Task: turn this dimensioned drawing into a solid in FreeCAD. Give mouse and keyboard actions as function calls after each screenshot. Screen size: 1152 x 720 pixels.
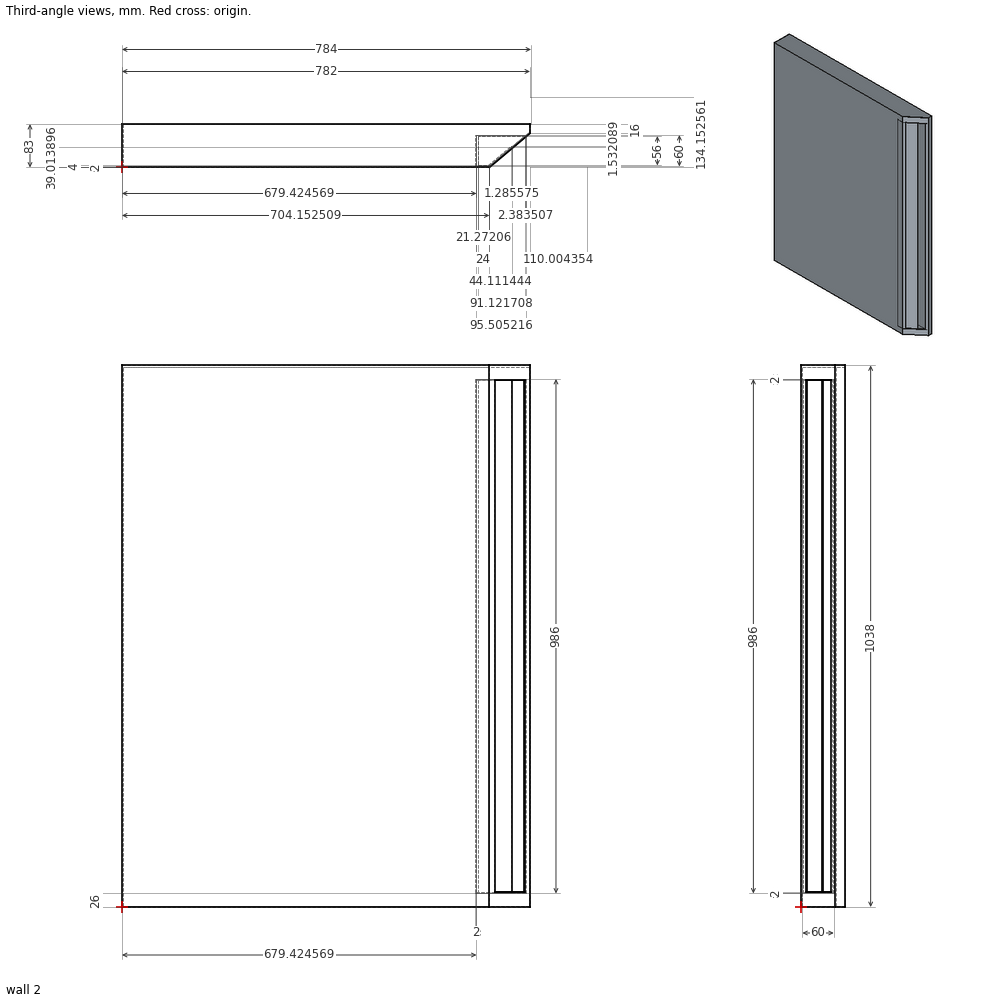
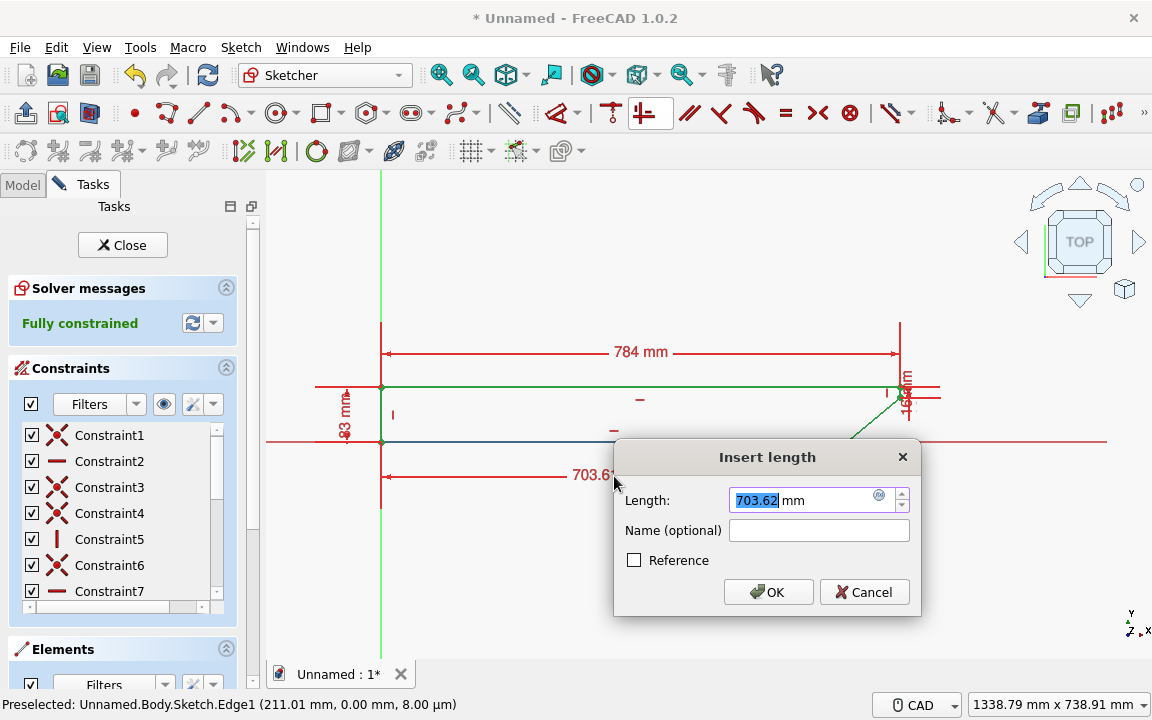
text(704.152509)
key(Return)
key(Escape)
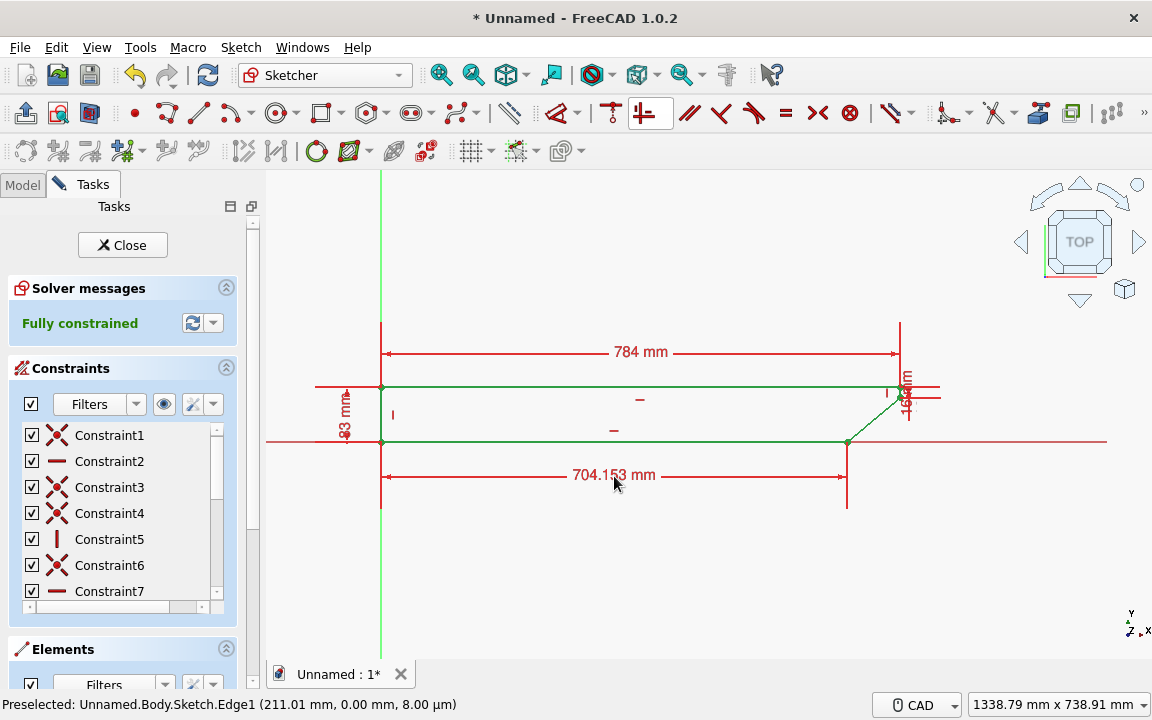
click(123, 245)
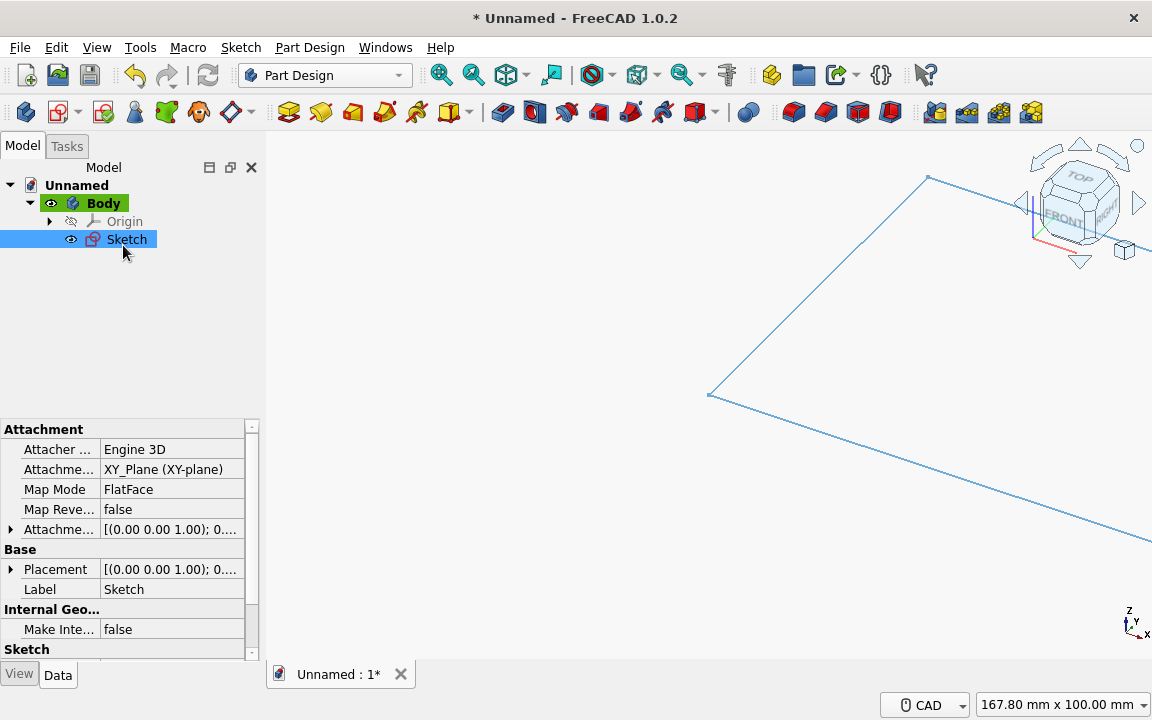
click(290, 112)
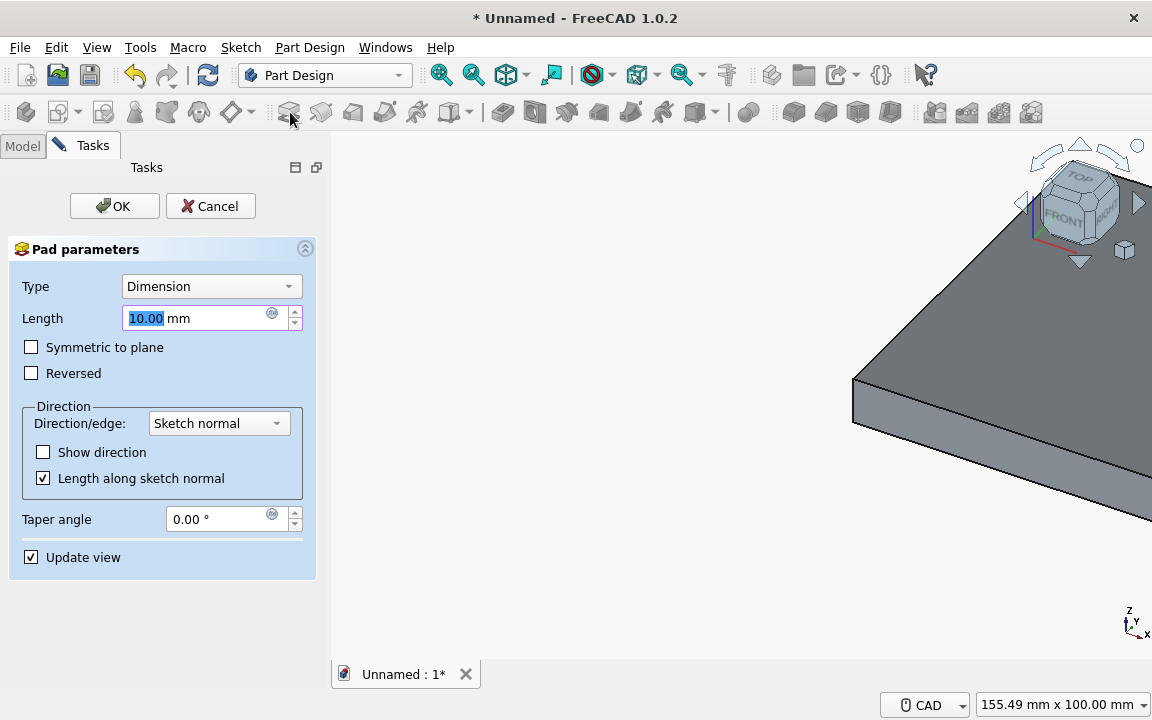
text(1038)
key(Tab)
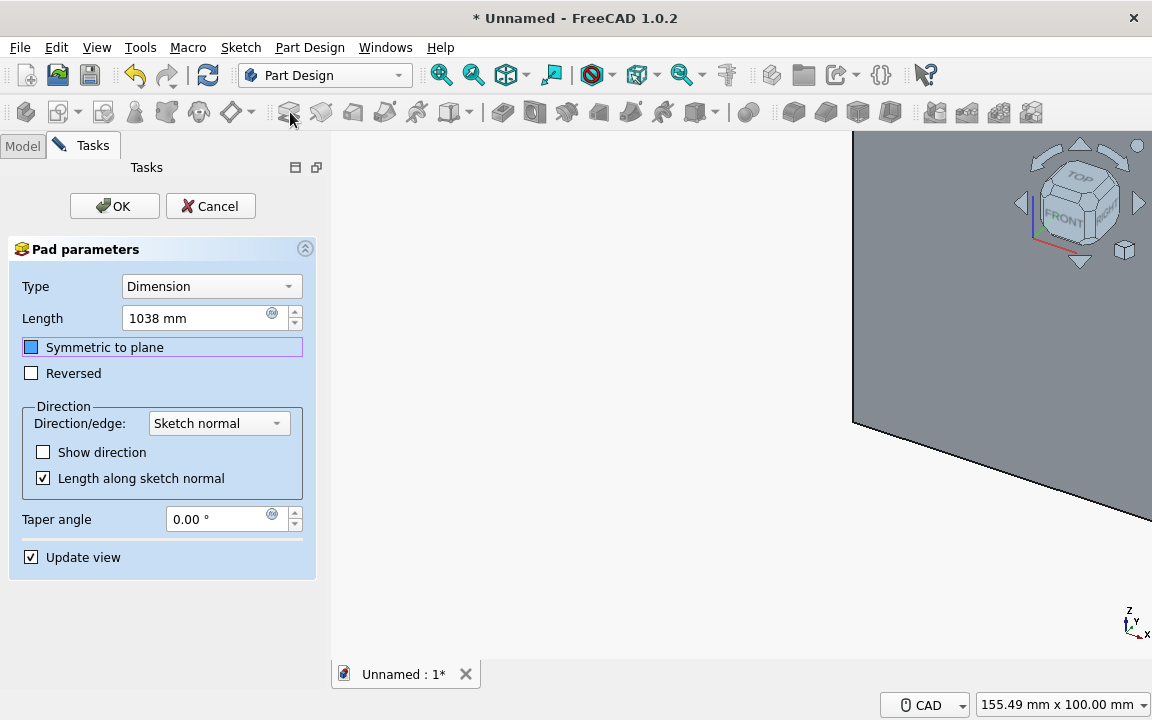
click(115, 206)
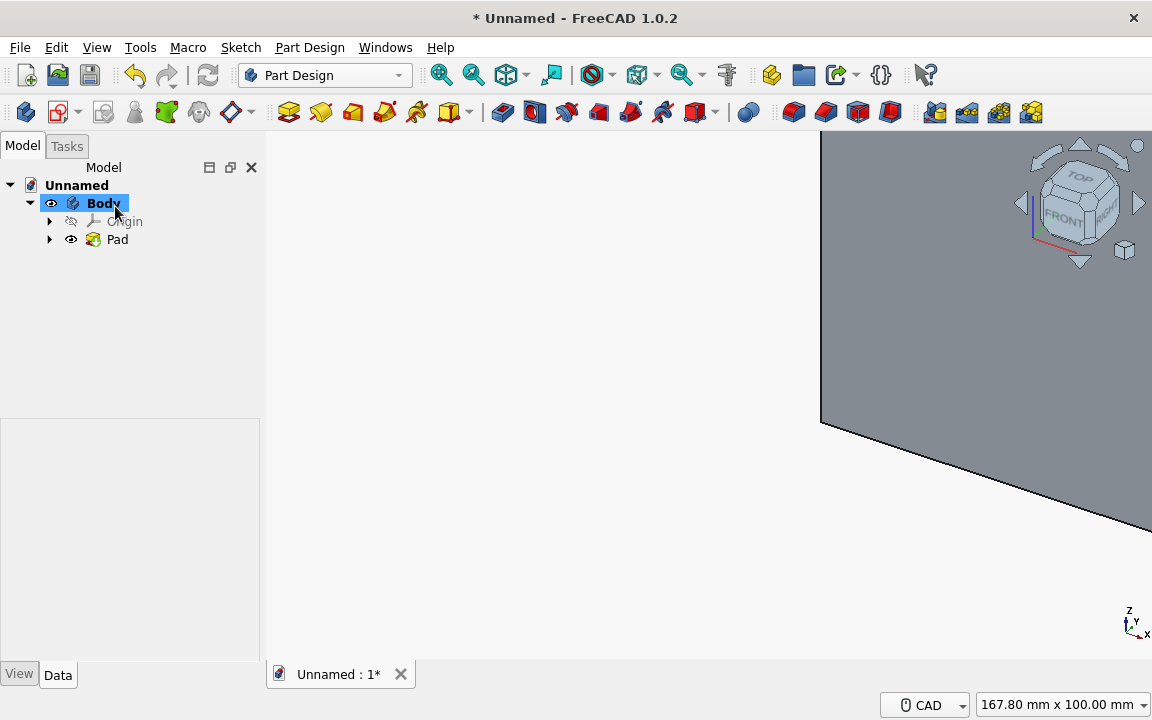
click(442, 76)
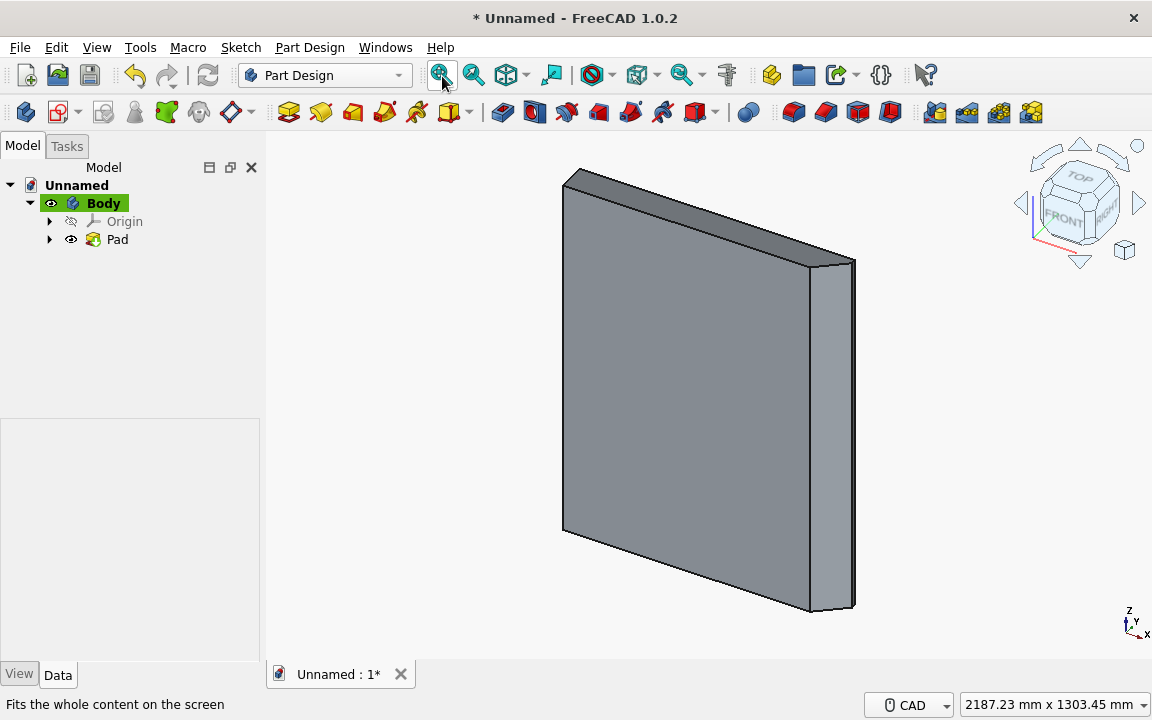
click(788, 248)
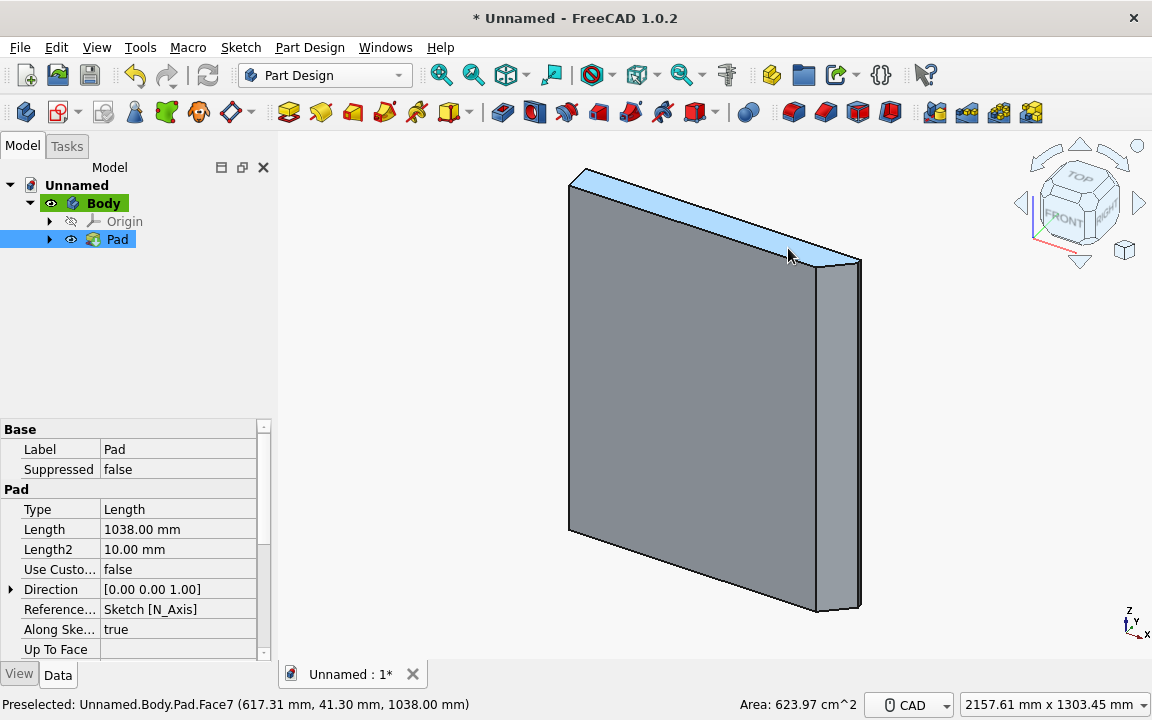
click(58, 112)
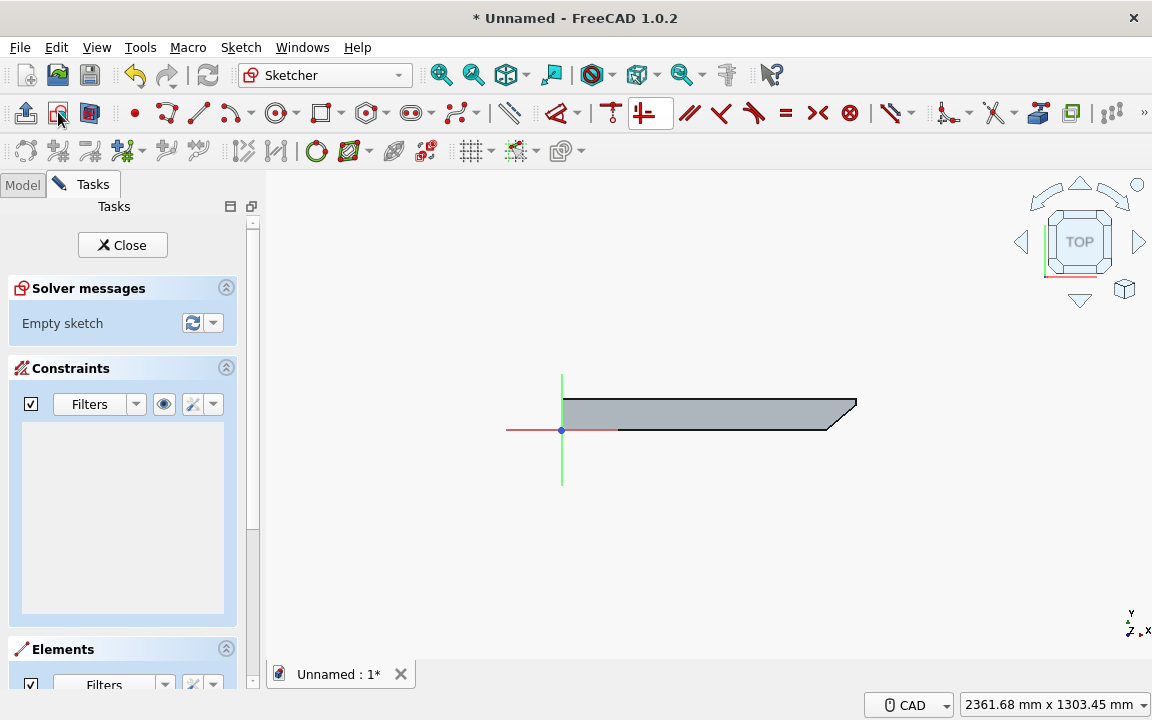
scroll(923, 403, up, 9)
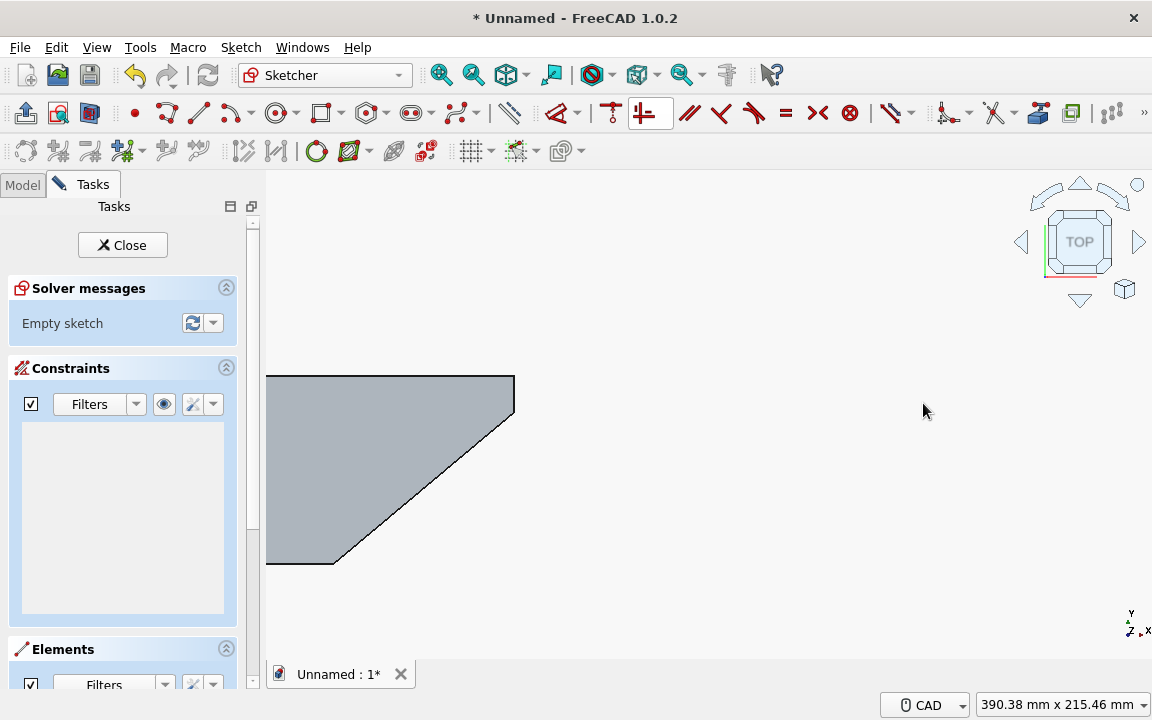
click(322, 114)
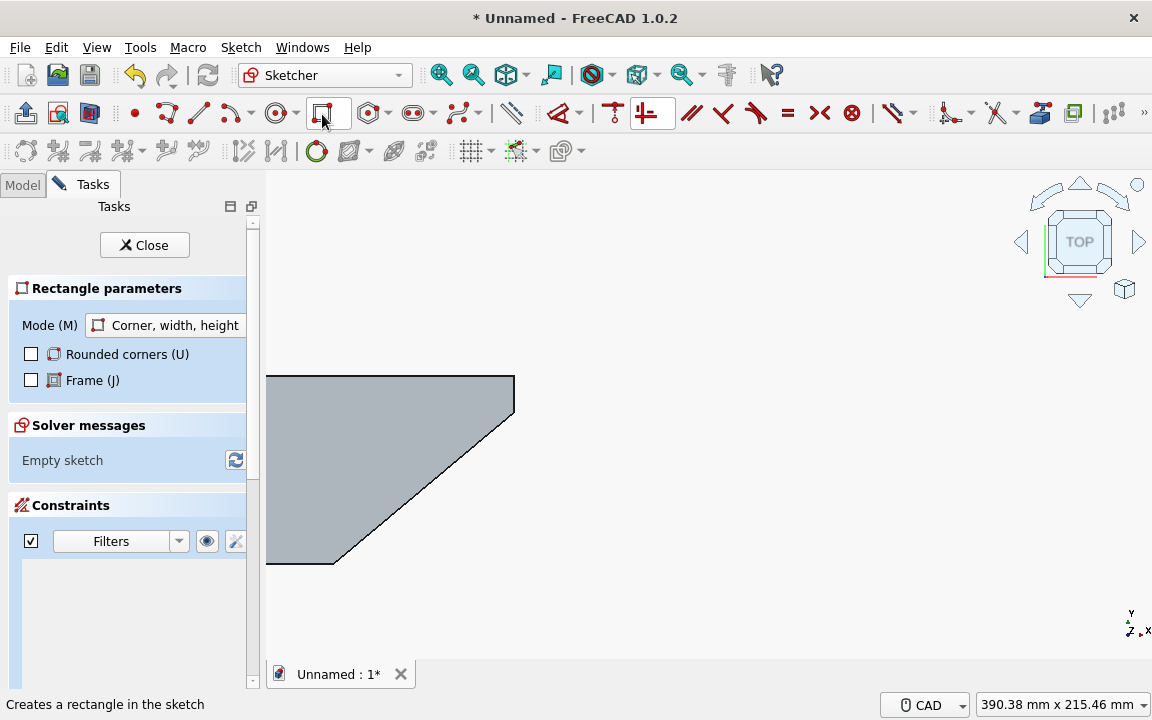
click(510, 260)
click(759, 564)
key(Escape)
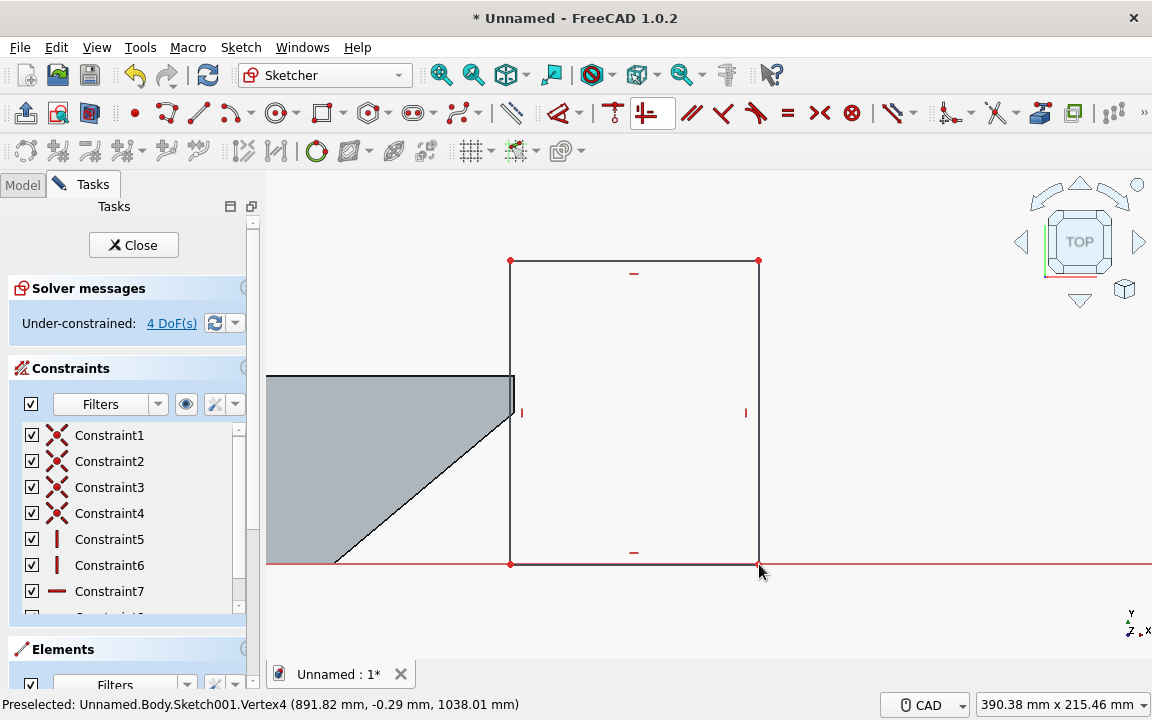
click(510, 565)